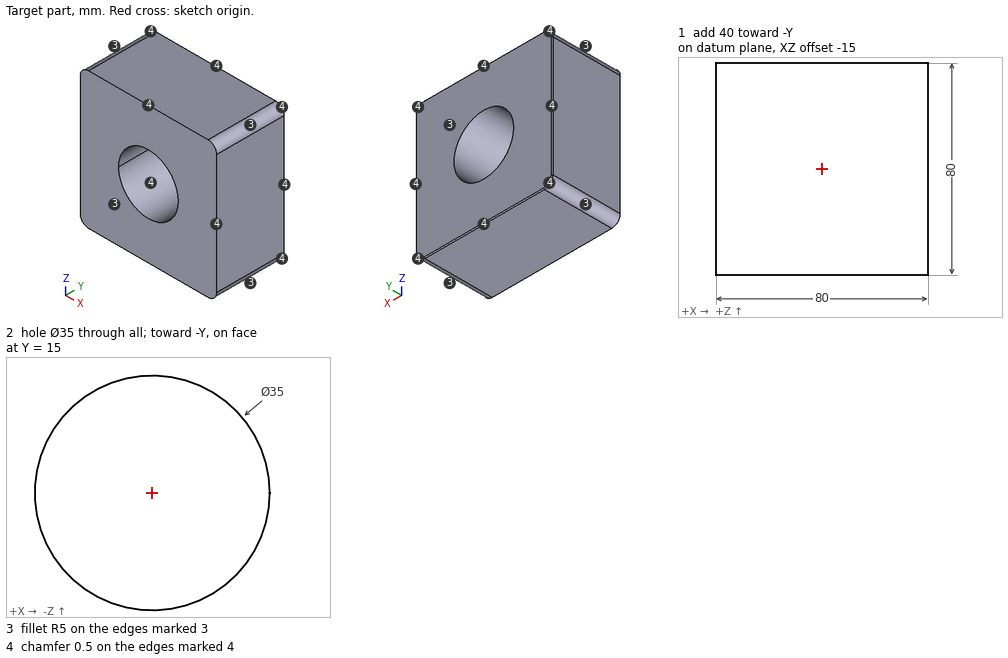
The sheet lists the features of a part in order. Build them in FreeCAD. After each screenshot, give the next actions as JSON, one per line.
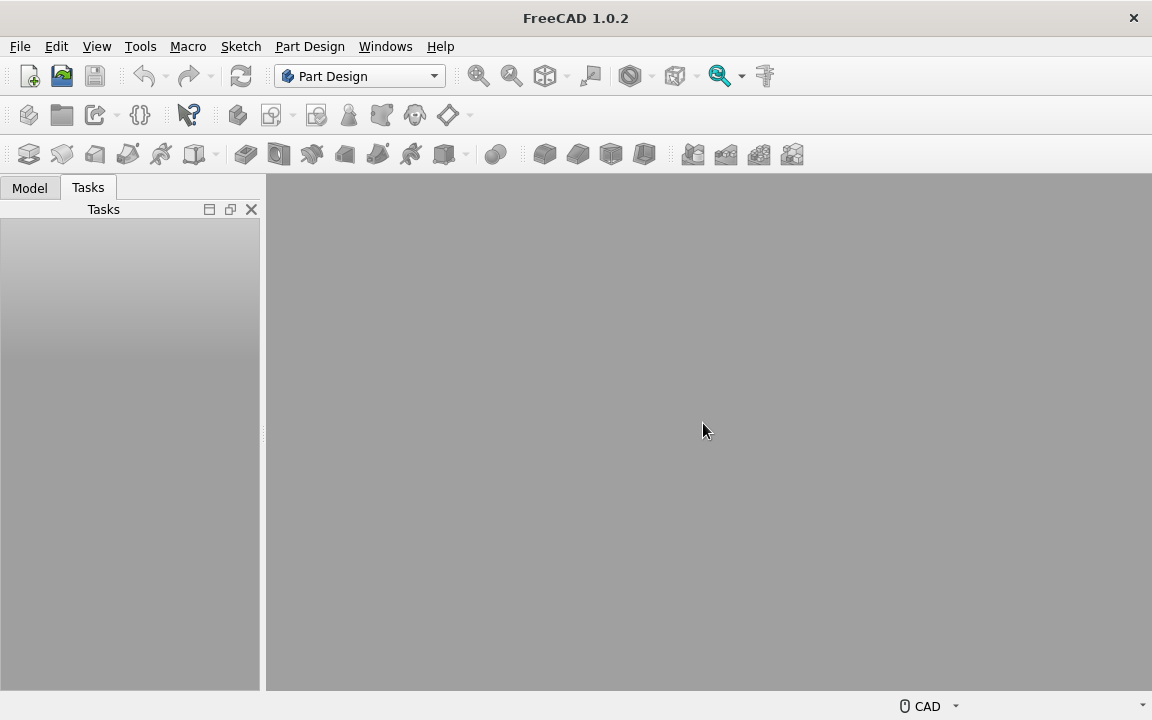
{"action": "left_click", "coordinate": [29, 76]}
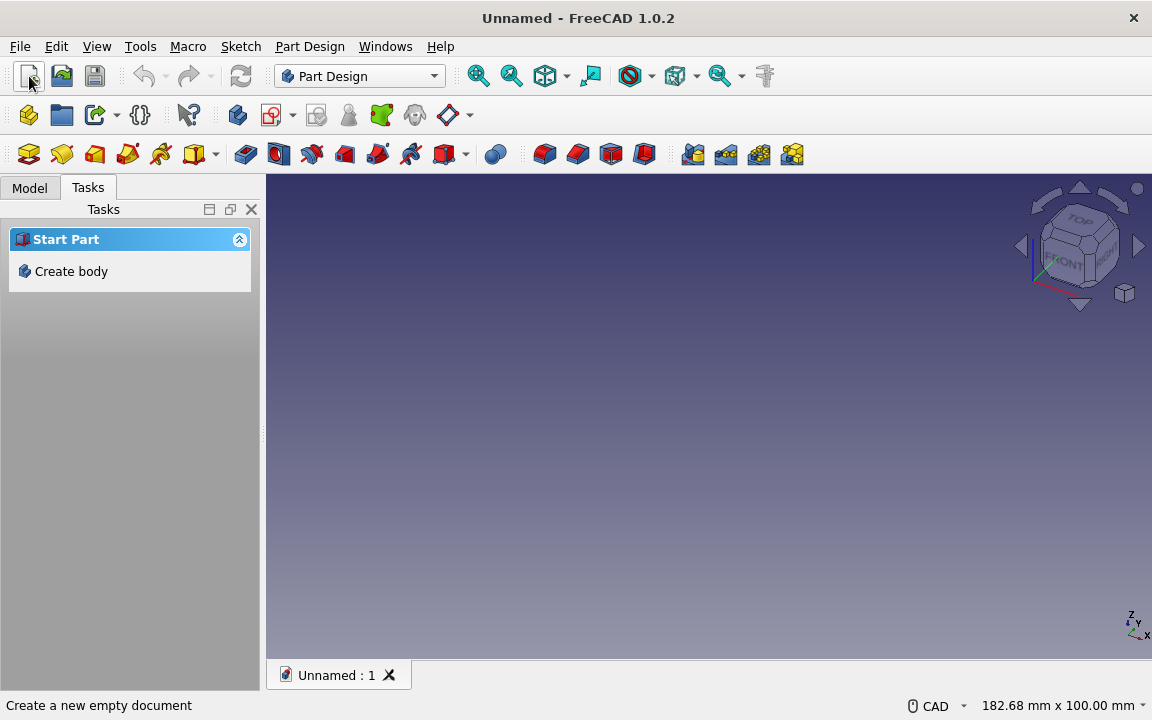
{"action": "left_click", "coordinate": [238, 116]}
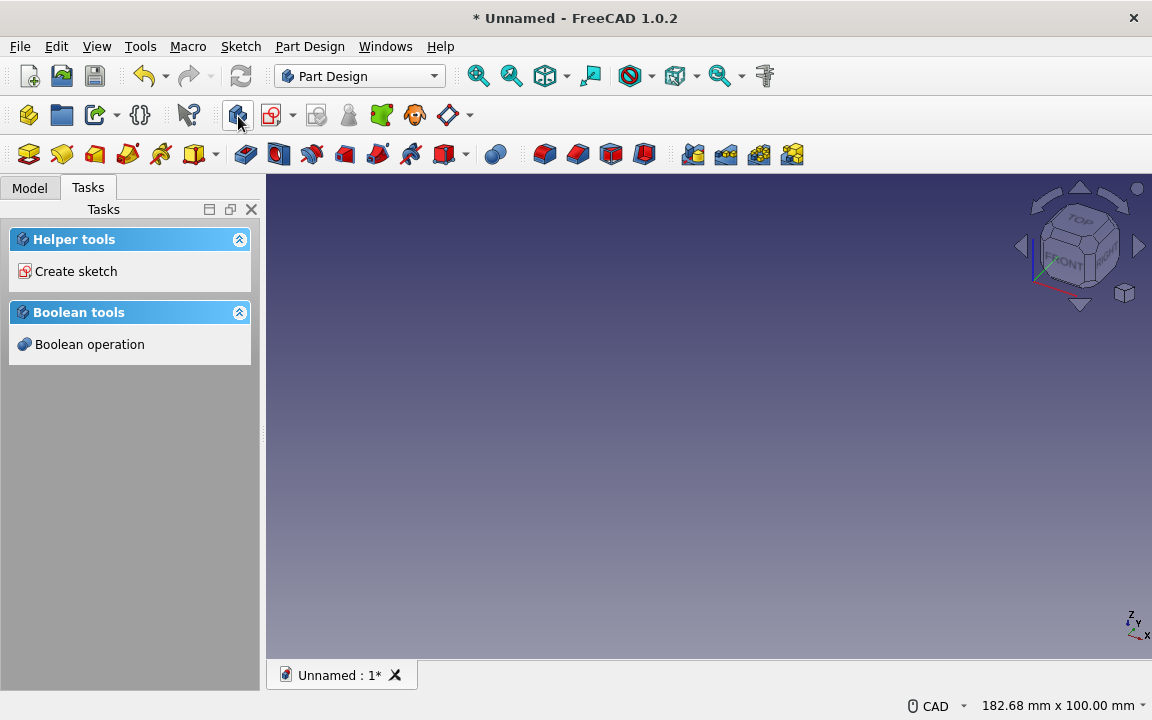
{"action": "left_click", "coordinate": [30, 188]}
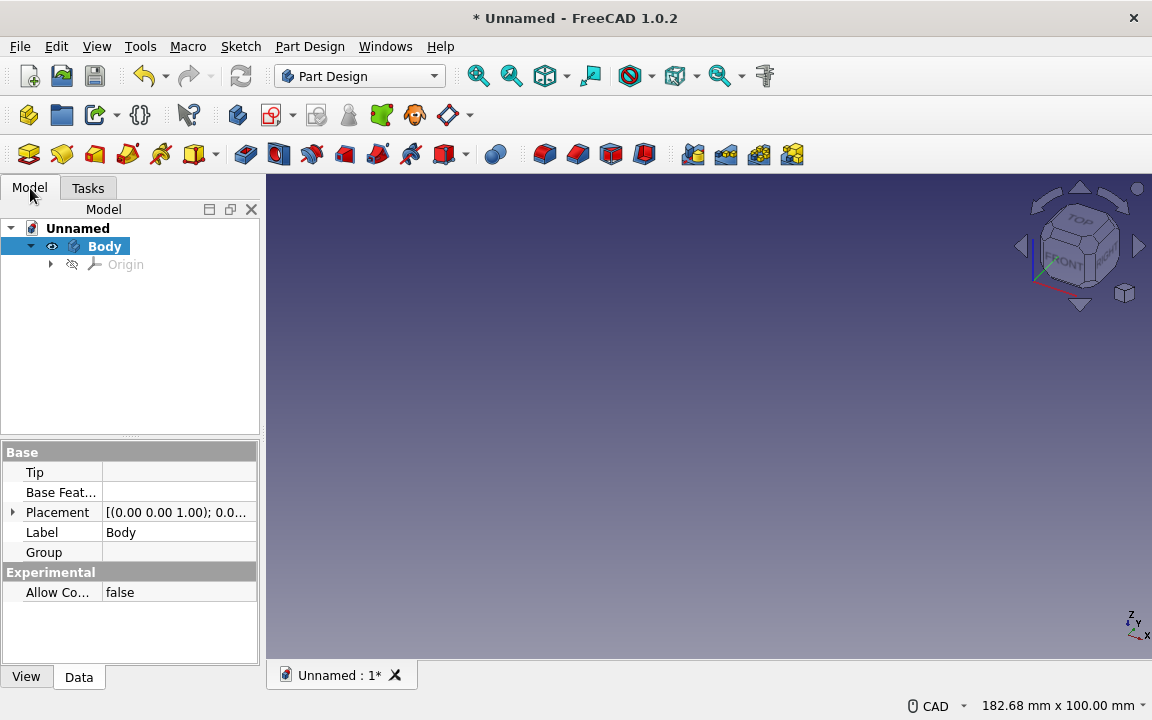
{"action": "left_click", "coordinate": [51, 264]}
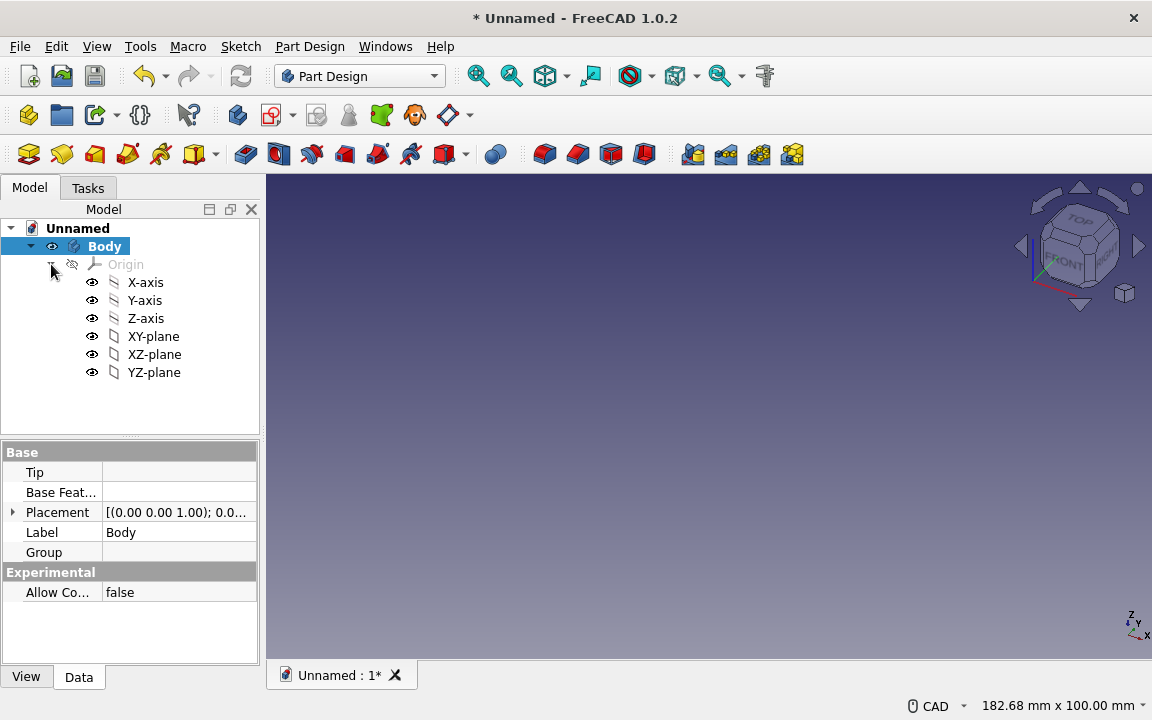
{"action": "left_click", "coordinate": [137, 354]}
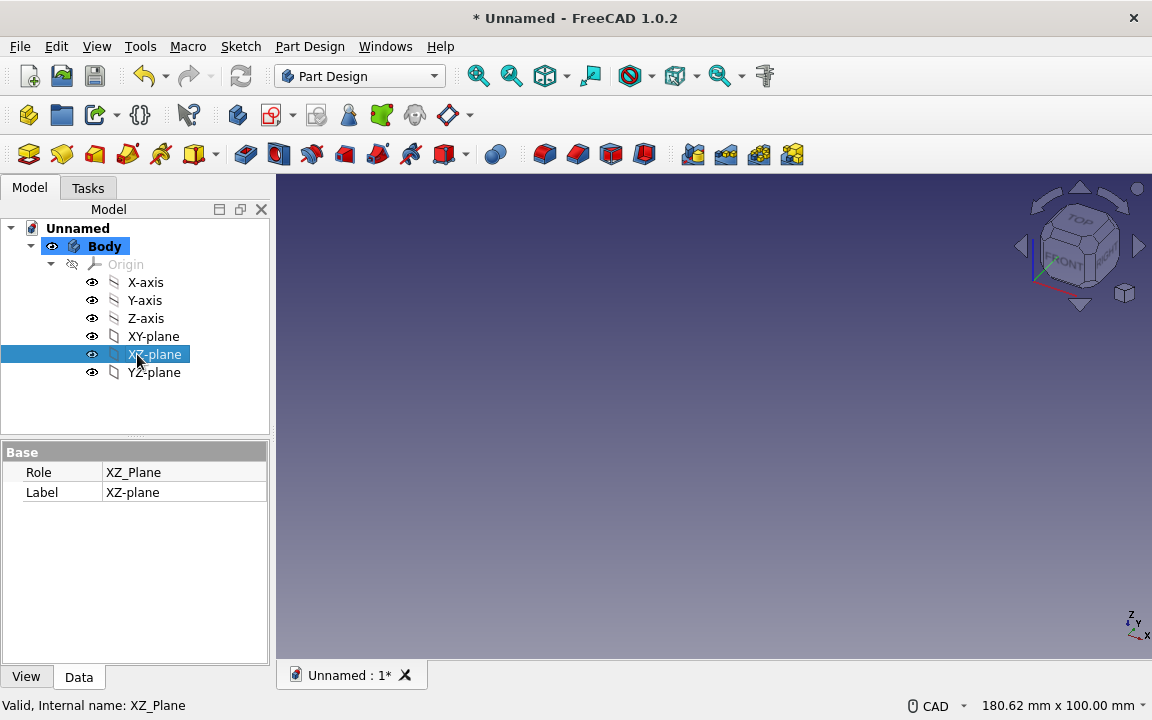
{"action": "left_click", "coordinate": [448, 116]}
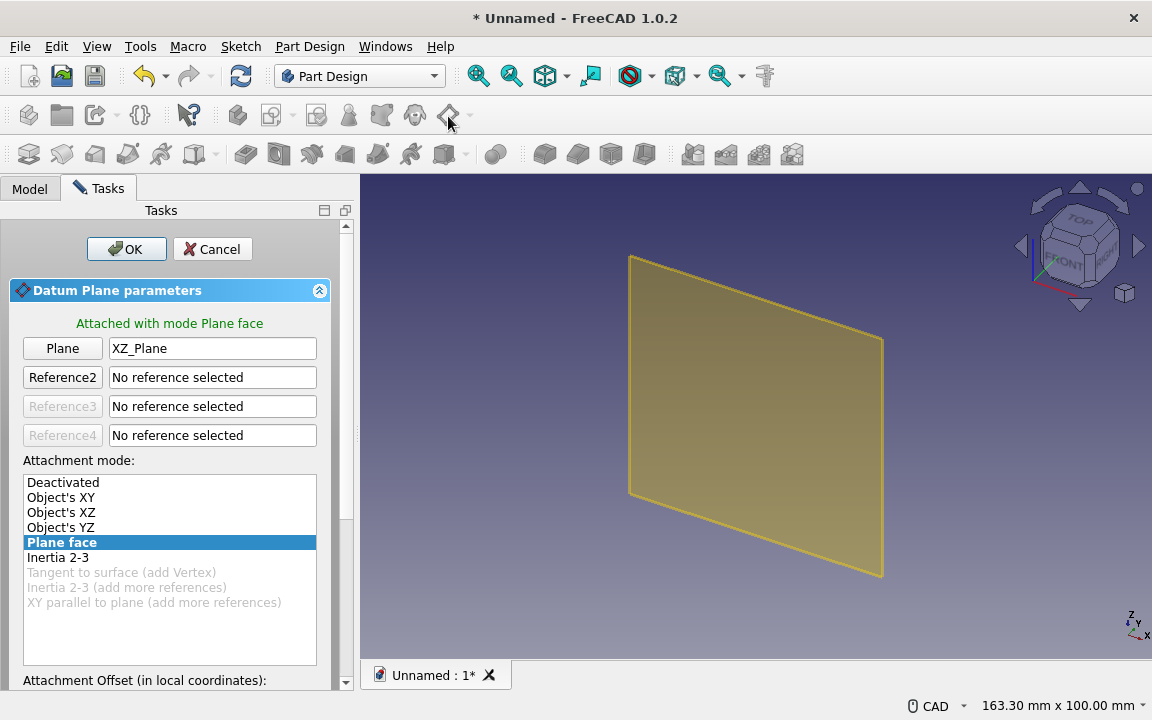
{"action": "scroll", "coordinate": [346, 455], "scroll_direction": "down", "scroll_amount": 3}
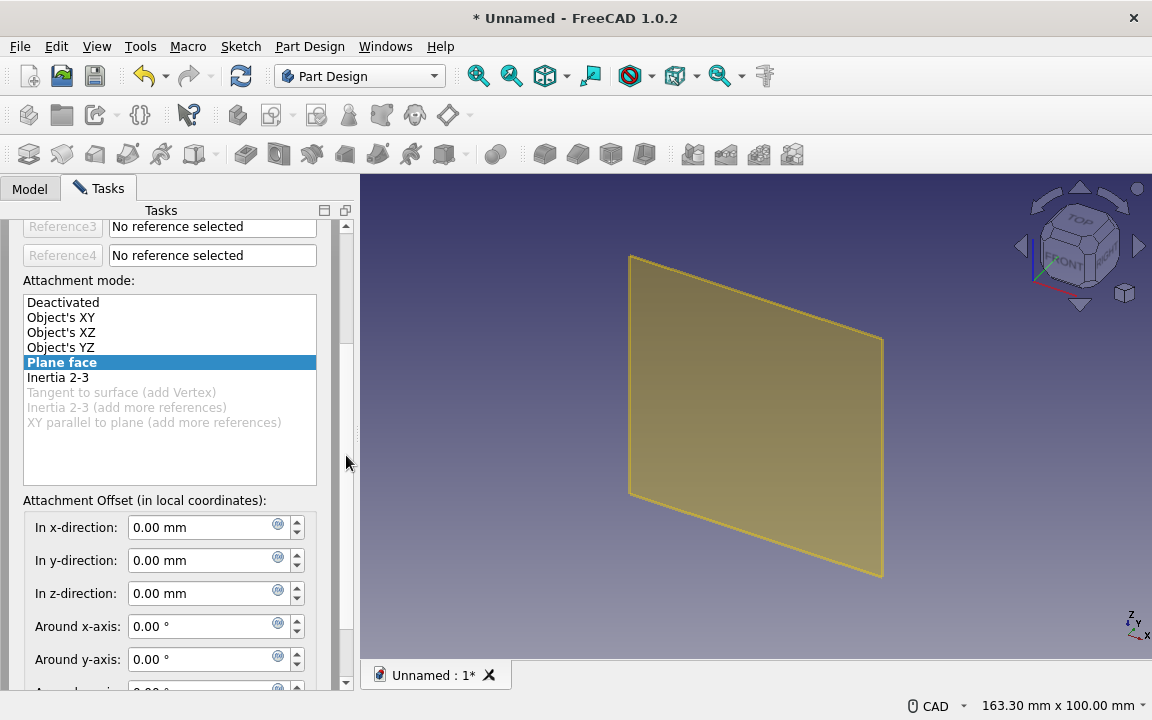
{"action": "triple_click", "coordinate": [210, 594]}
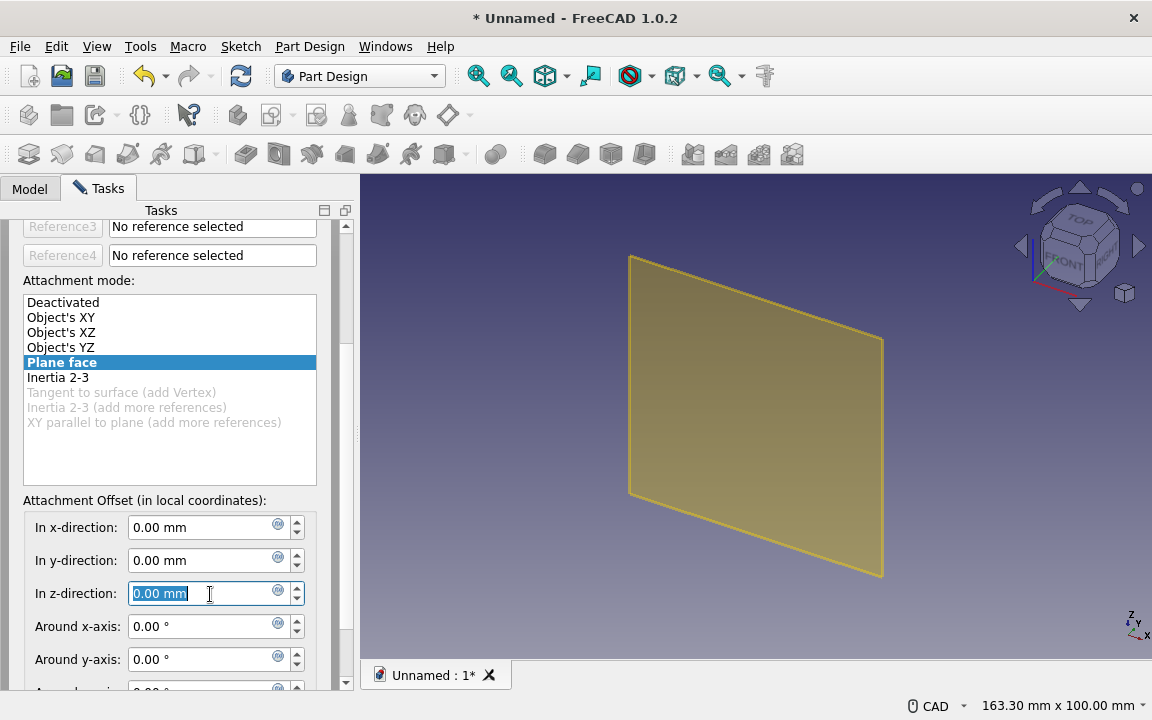
{"action": "type", "text": "-15"}
{"action": "key", "text": "Tab"}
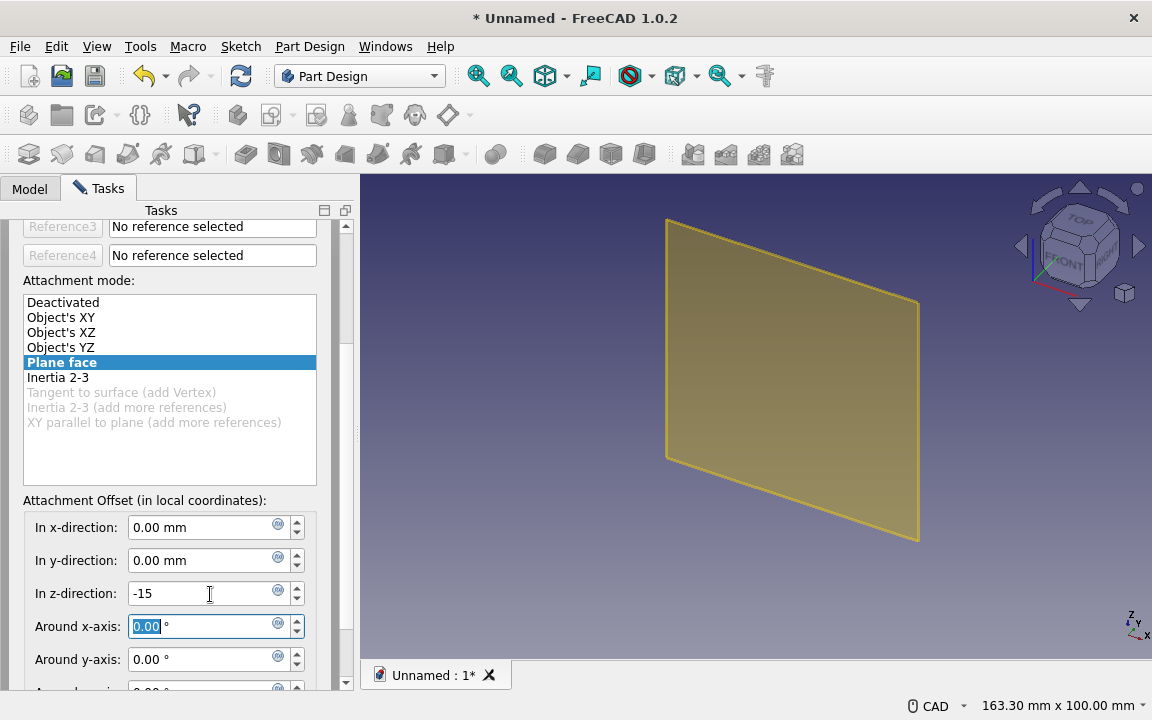
{"action": "scroll", "coordinate": [346, 455], "scroll_direction": "up", "scroll_amount": 4}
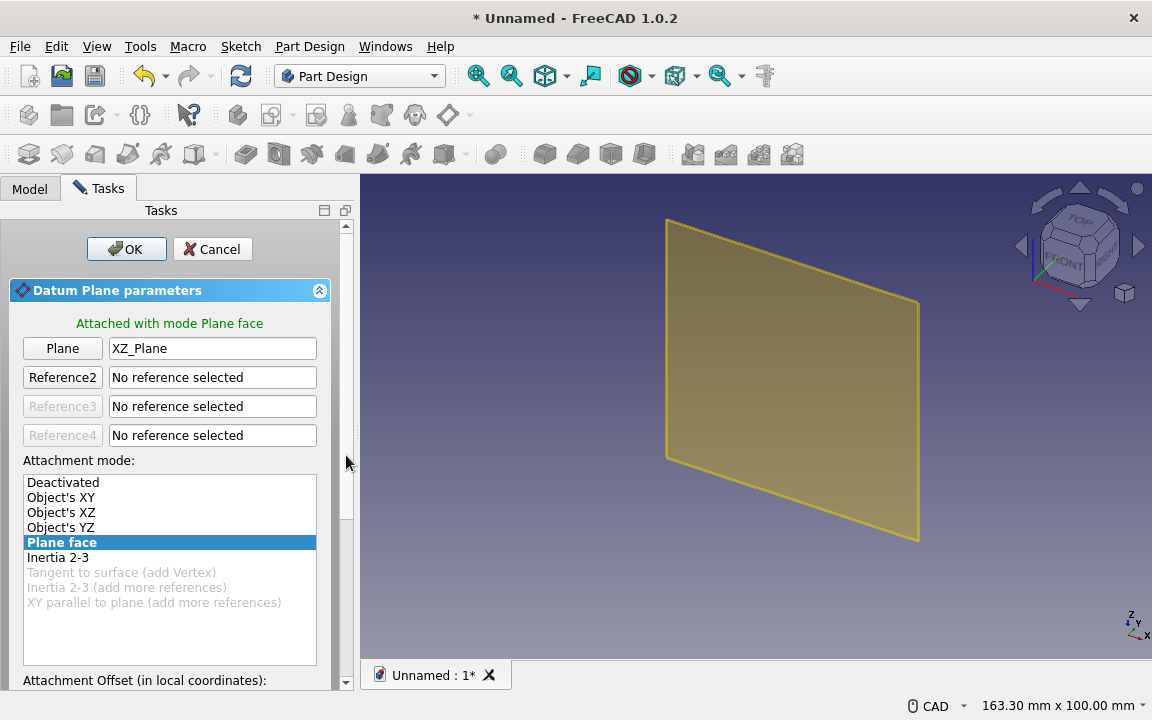
{"action": "left_click", "coordinate": [127, 249]}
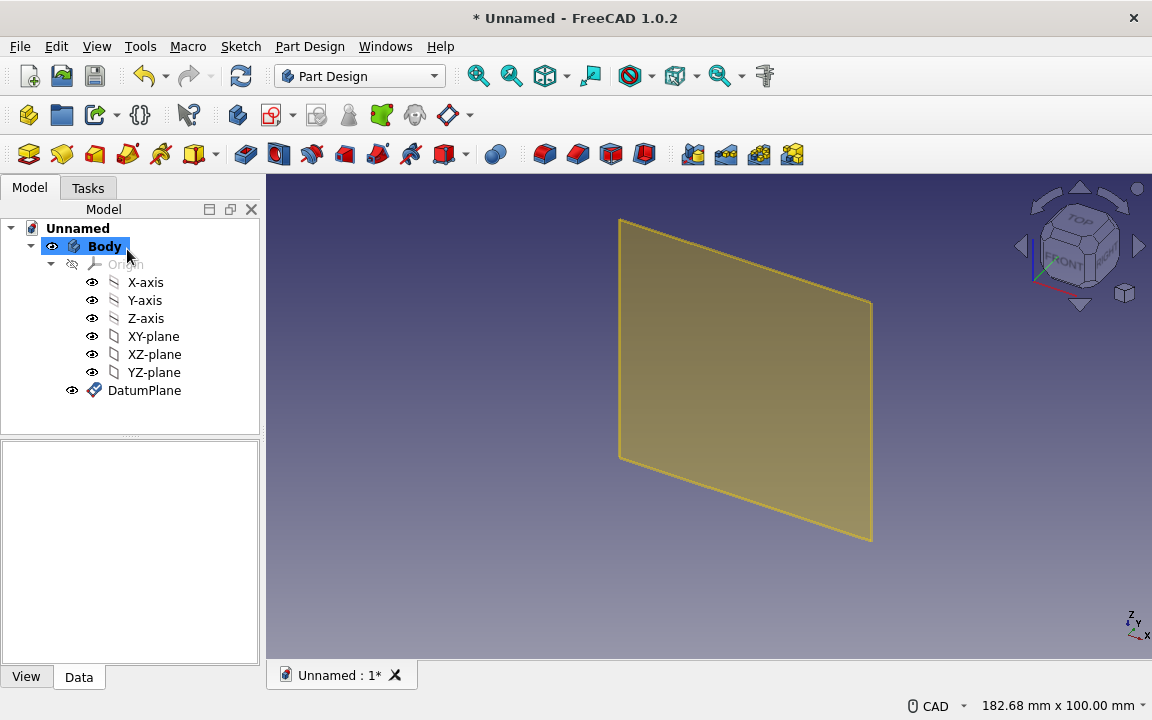
{"action": "left_click", "coordinate": [117, 390]}